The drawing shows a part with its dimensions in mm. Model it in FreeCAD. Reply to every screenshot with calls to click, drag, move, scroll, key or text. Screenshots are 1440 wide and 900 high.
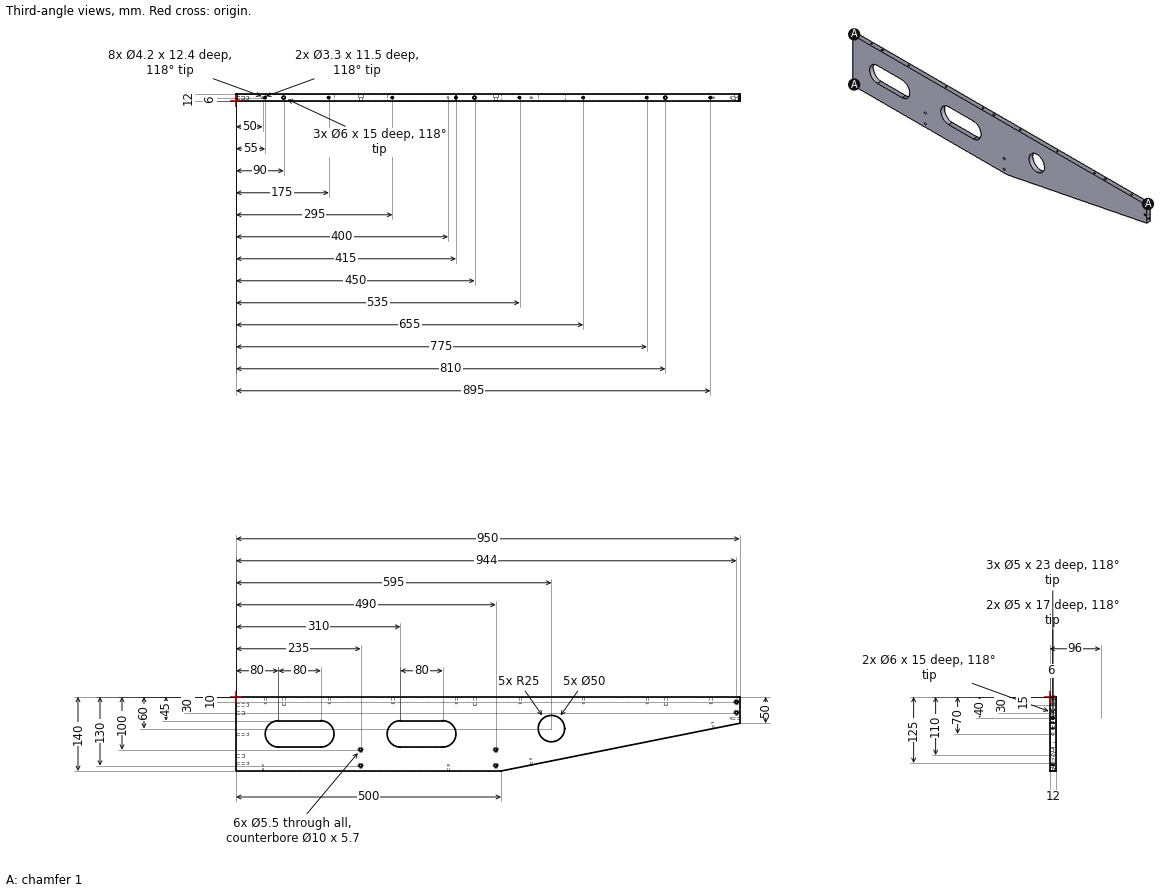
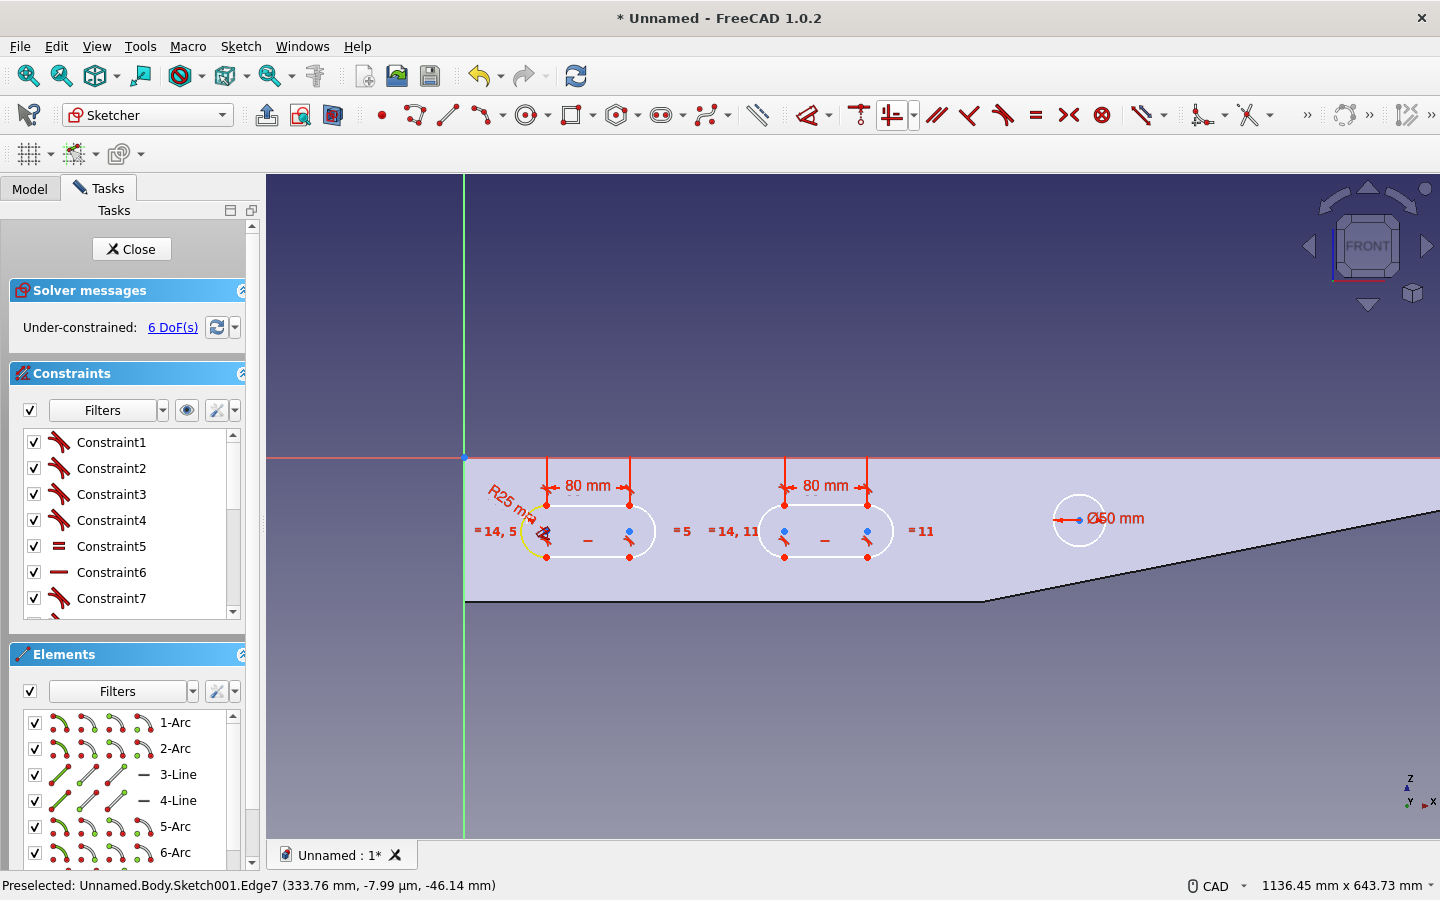
click(1079, 520)
click(430, 489)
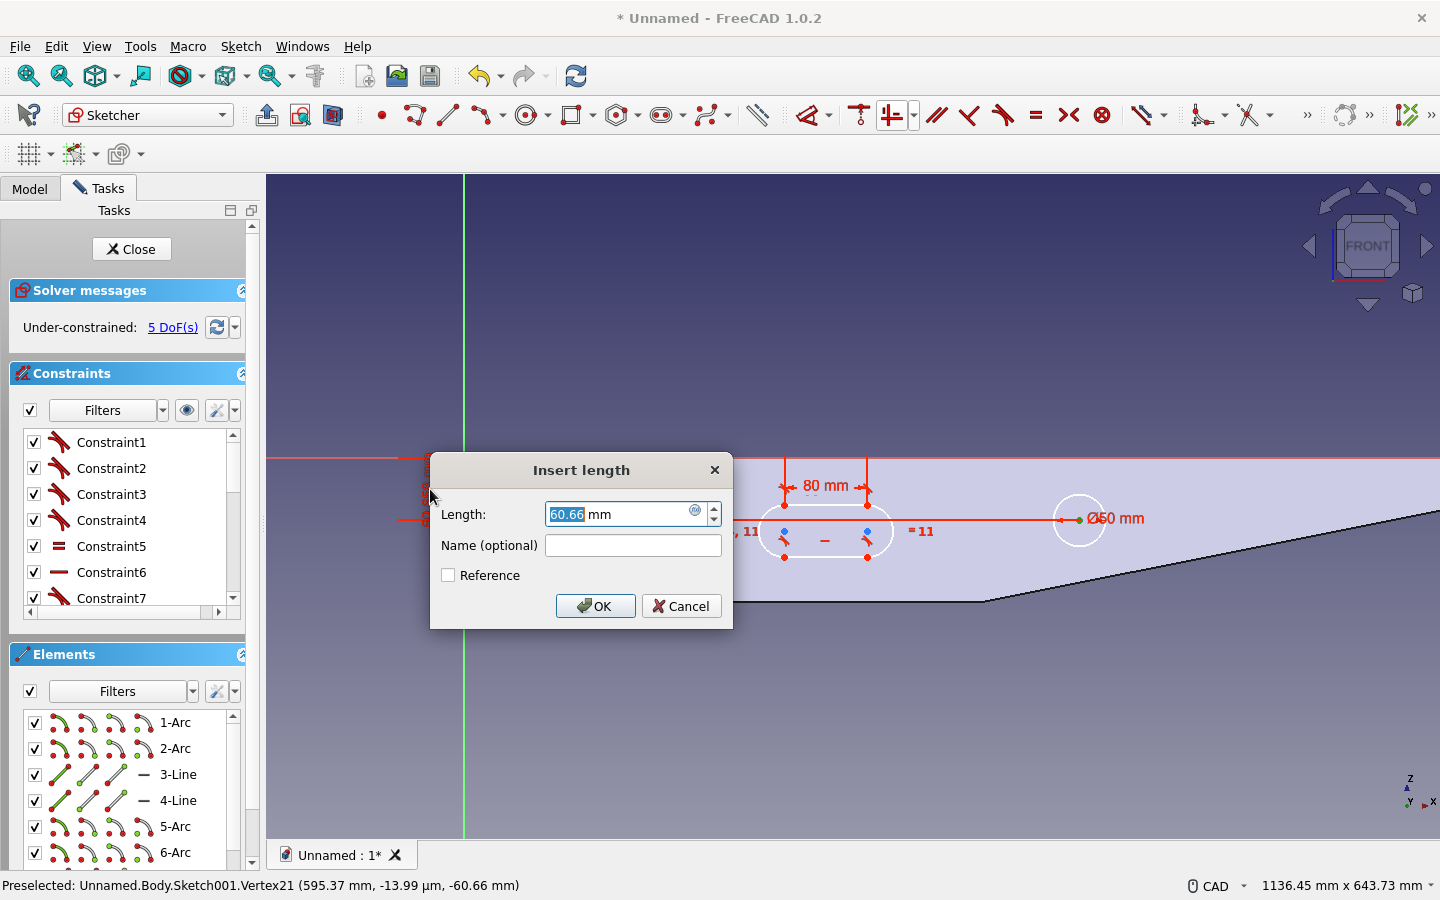
text(60)
key(Return)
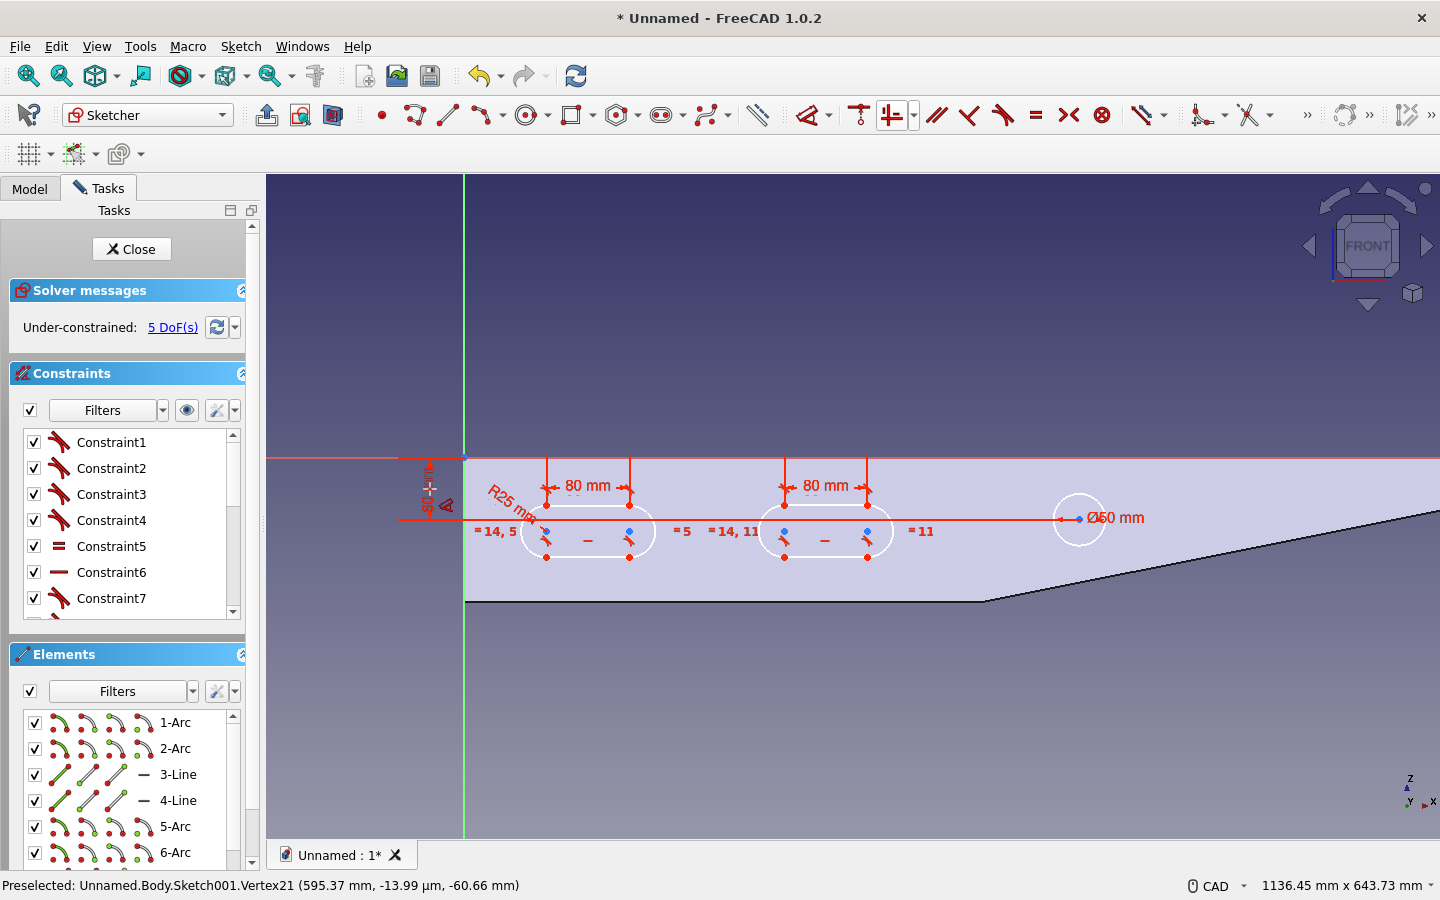
click(547, 506)
click(506, 424)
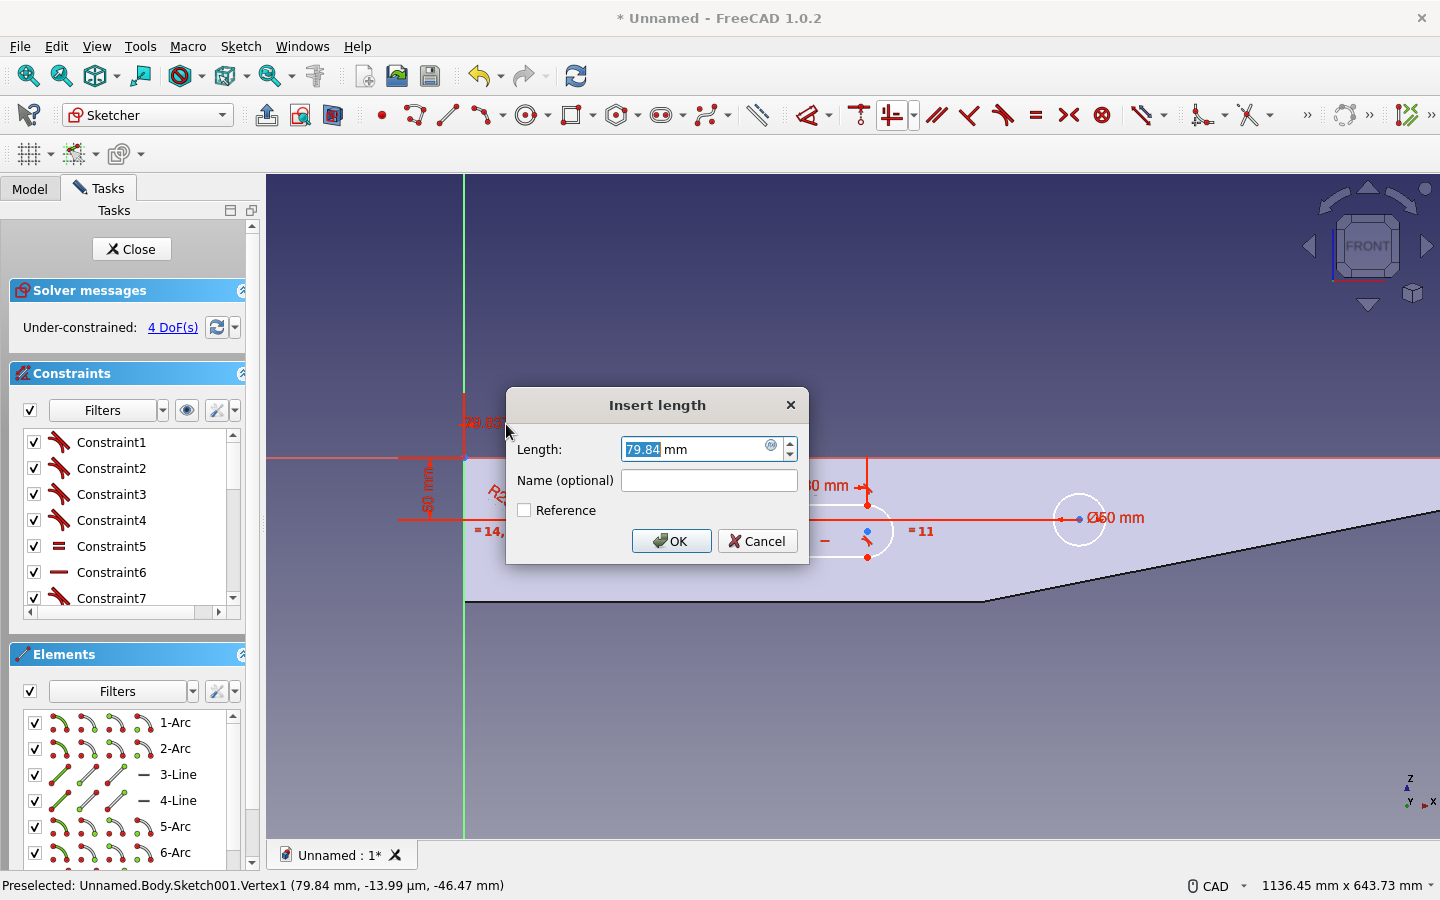
text(80)
key(Return)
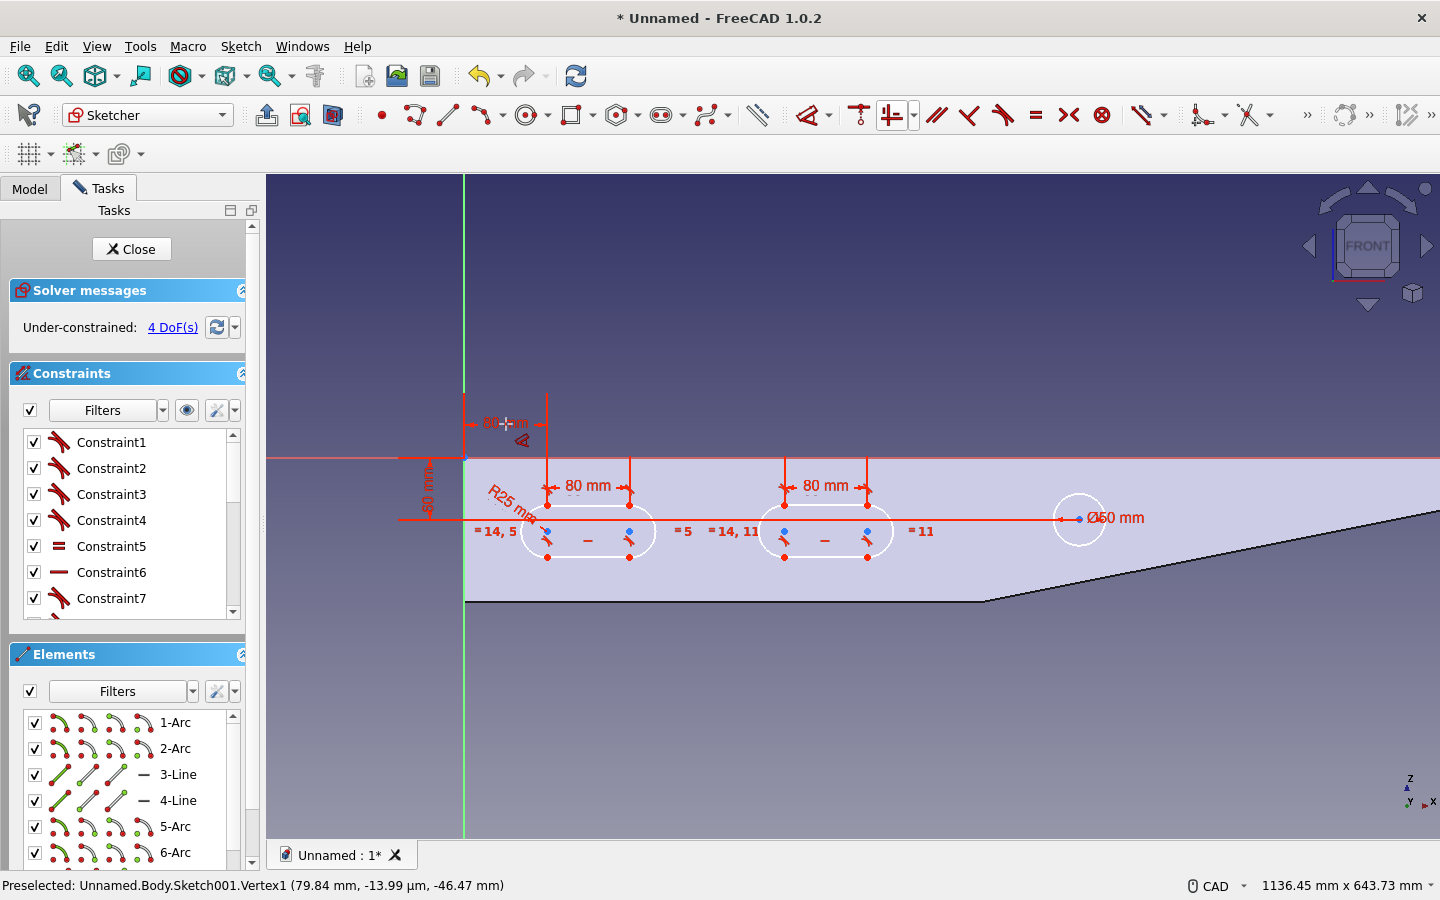
click(547, 506)
click(358, 482)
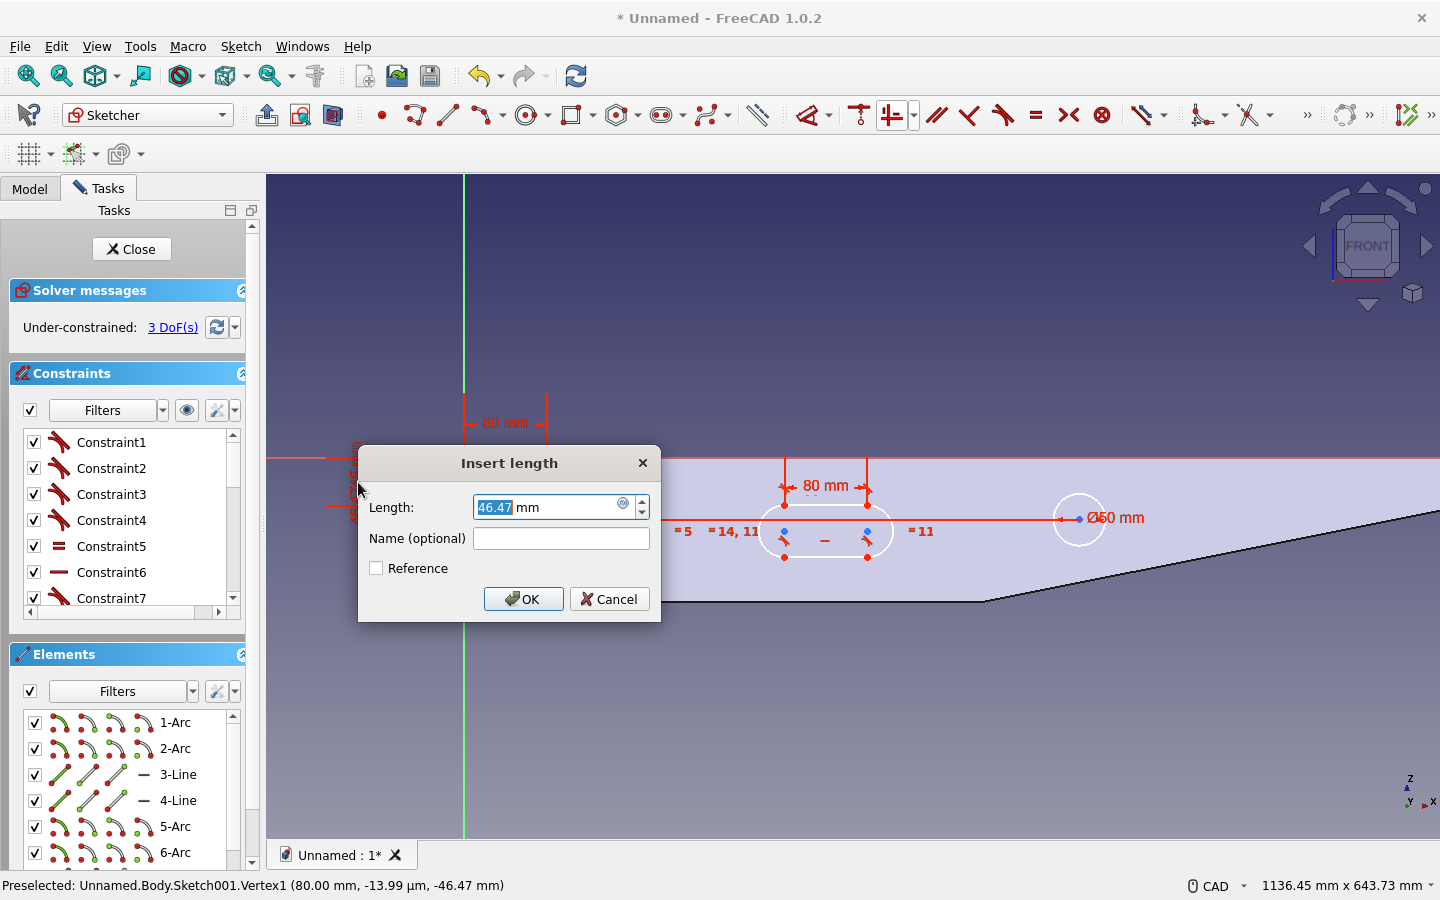
text(45)
key(Return)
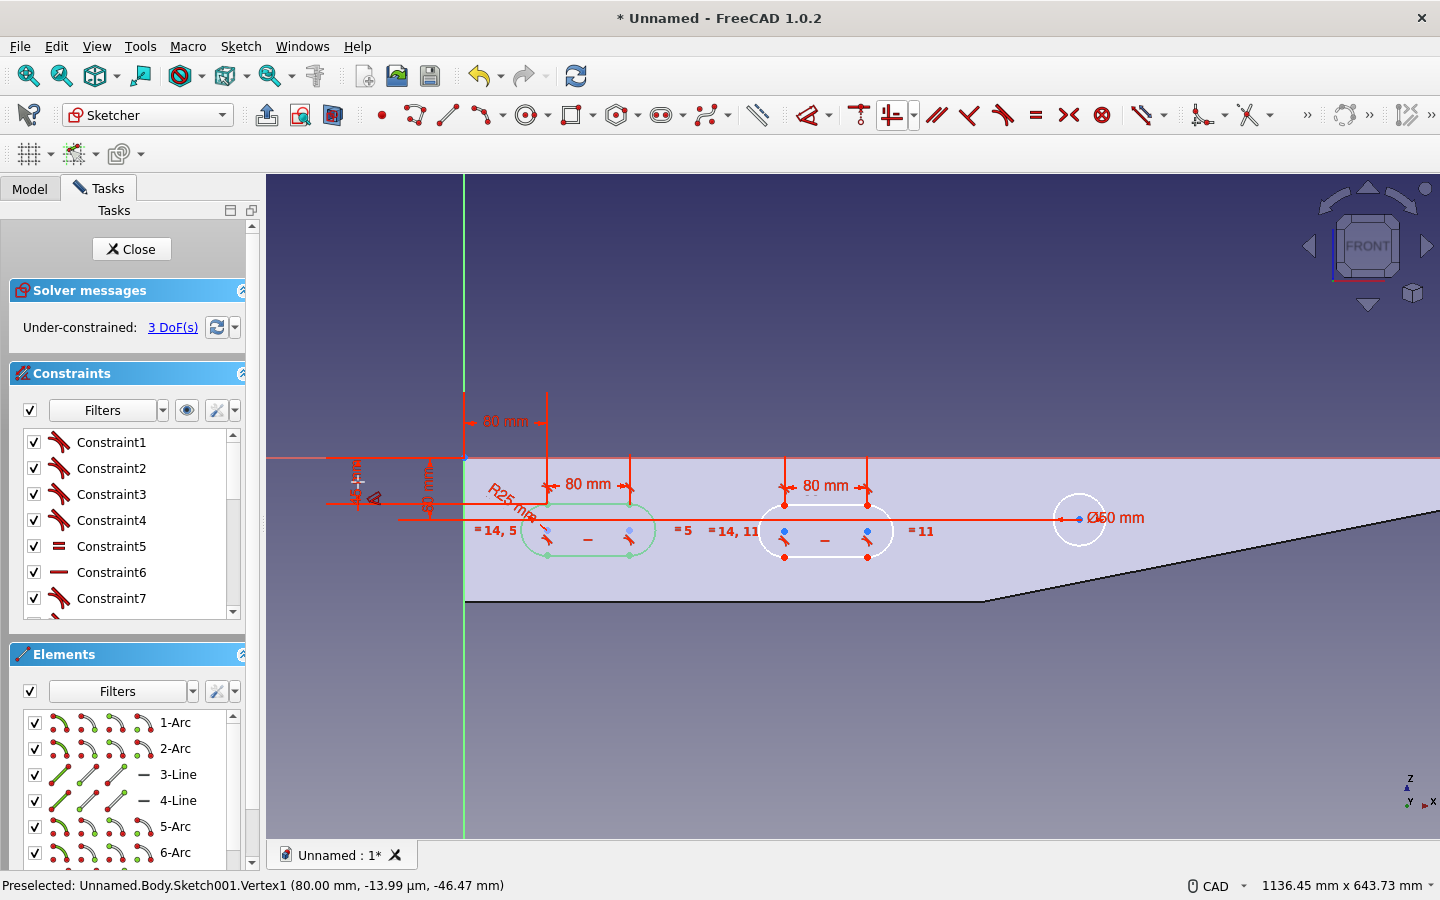
click(785, 505)
click(915, 482)